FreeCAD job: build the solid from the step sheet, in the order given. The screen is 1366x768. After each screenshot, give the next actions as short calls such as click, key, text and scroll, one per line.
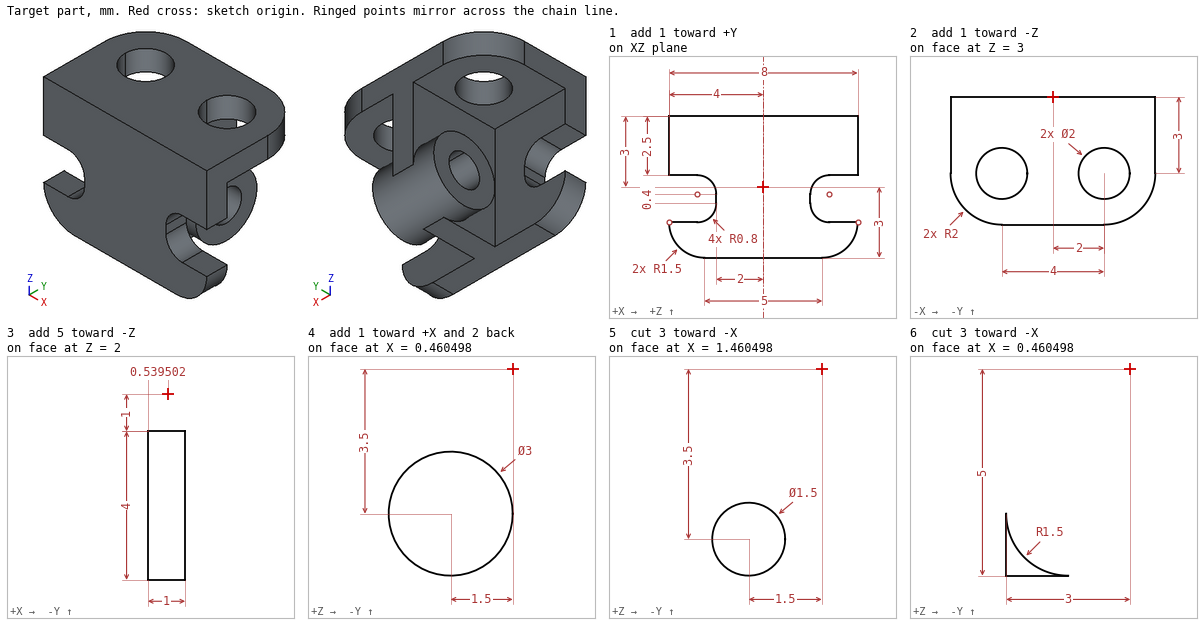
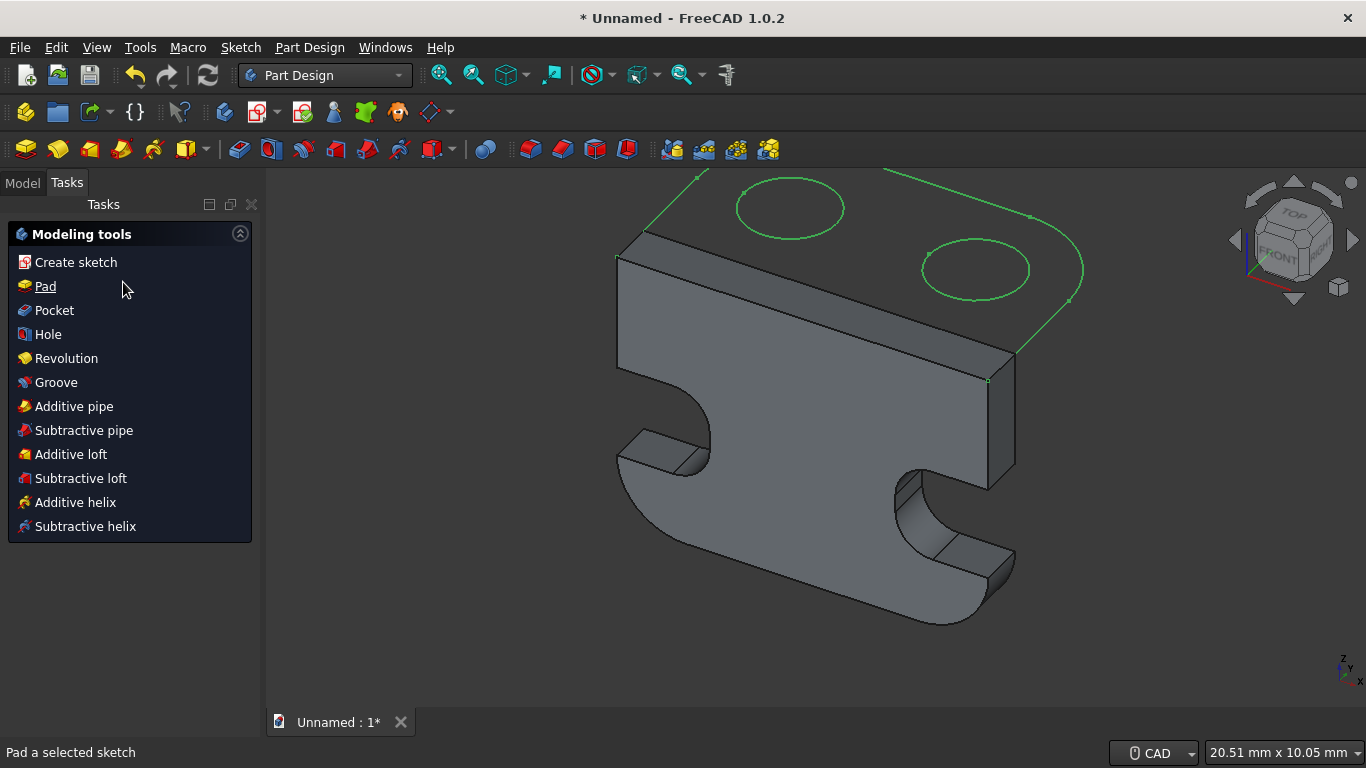
click(26, 150)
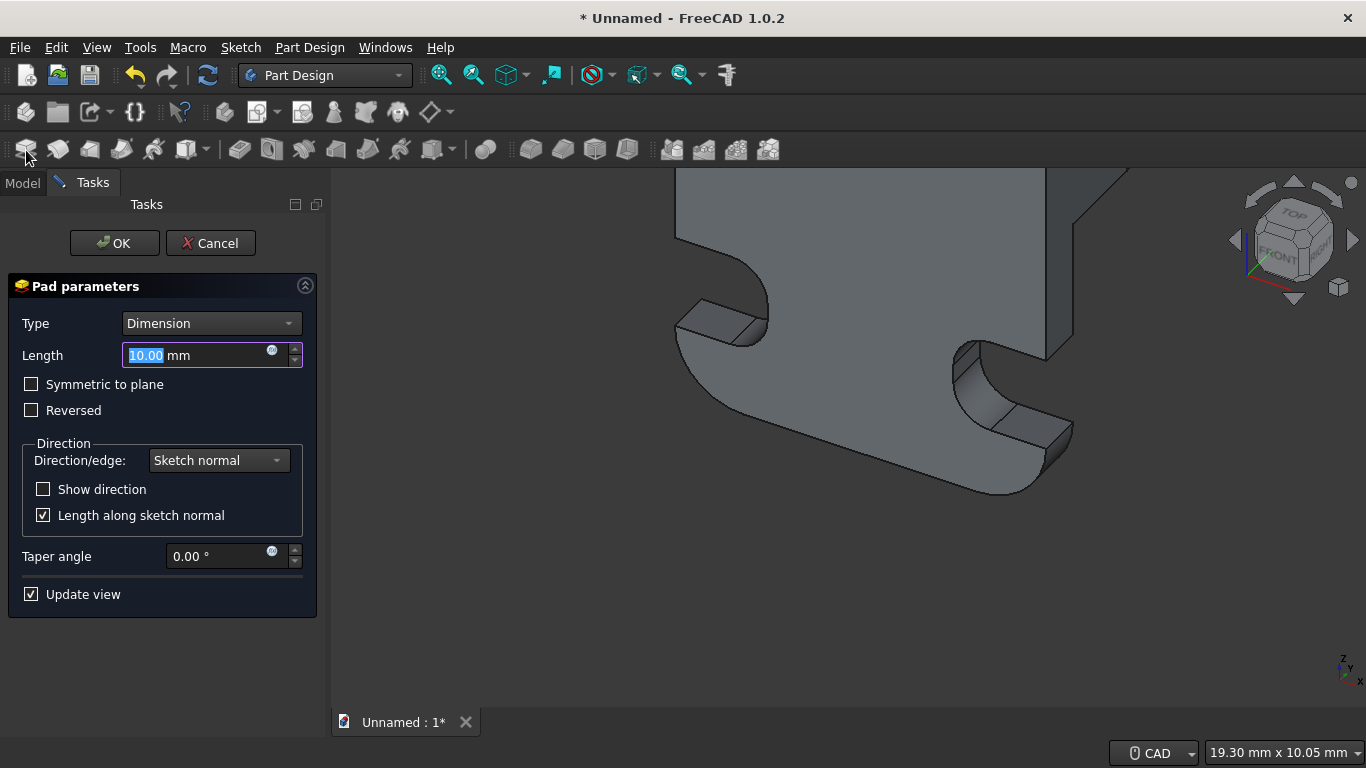
text(1)
key(Tab)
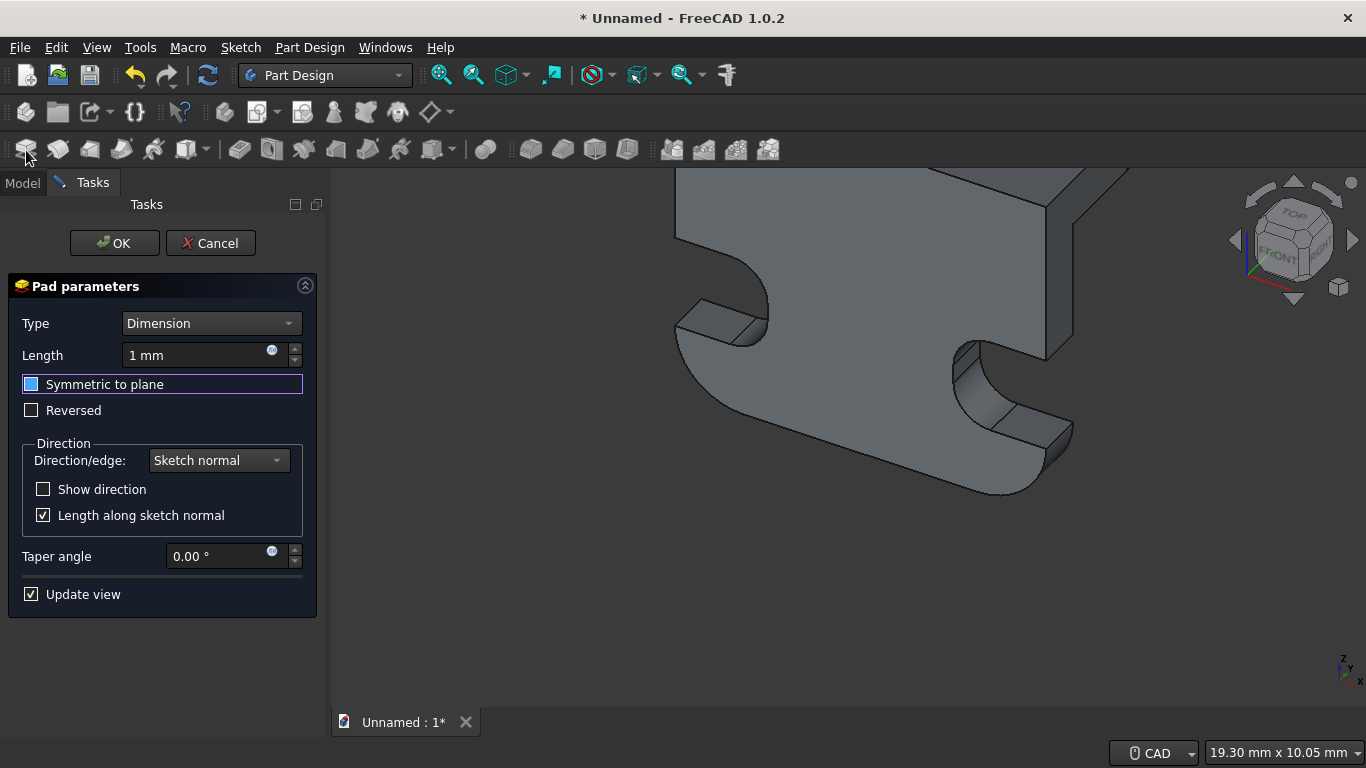
click(30, 410)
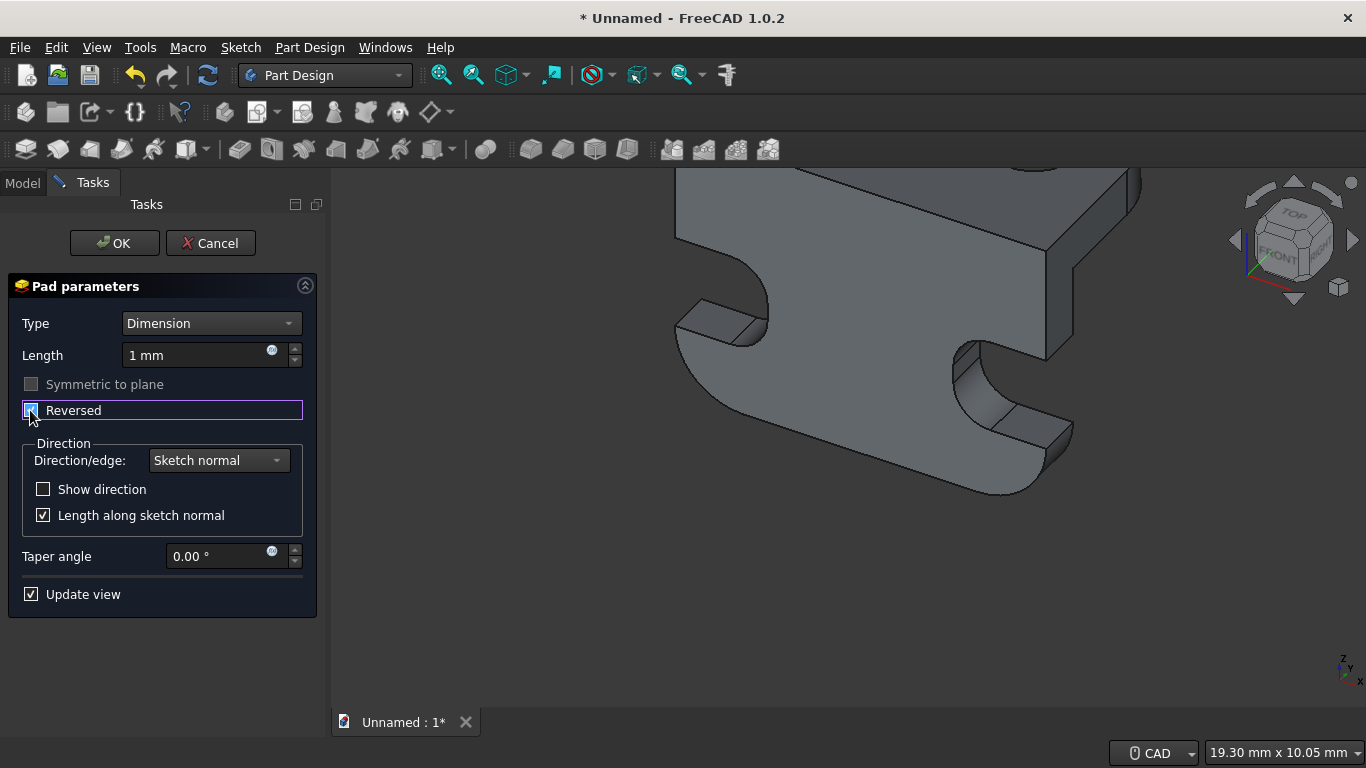
click(115, 243)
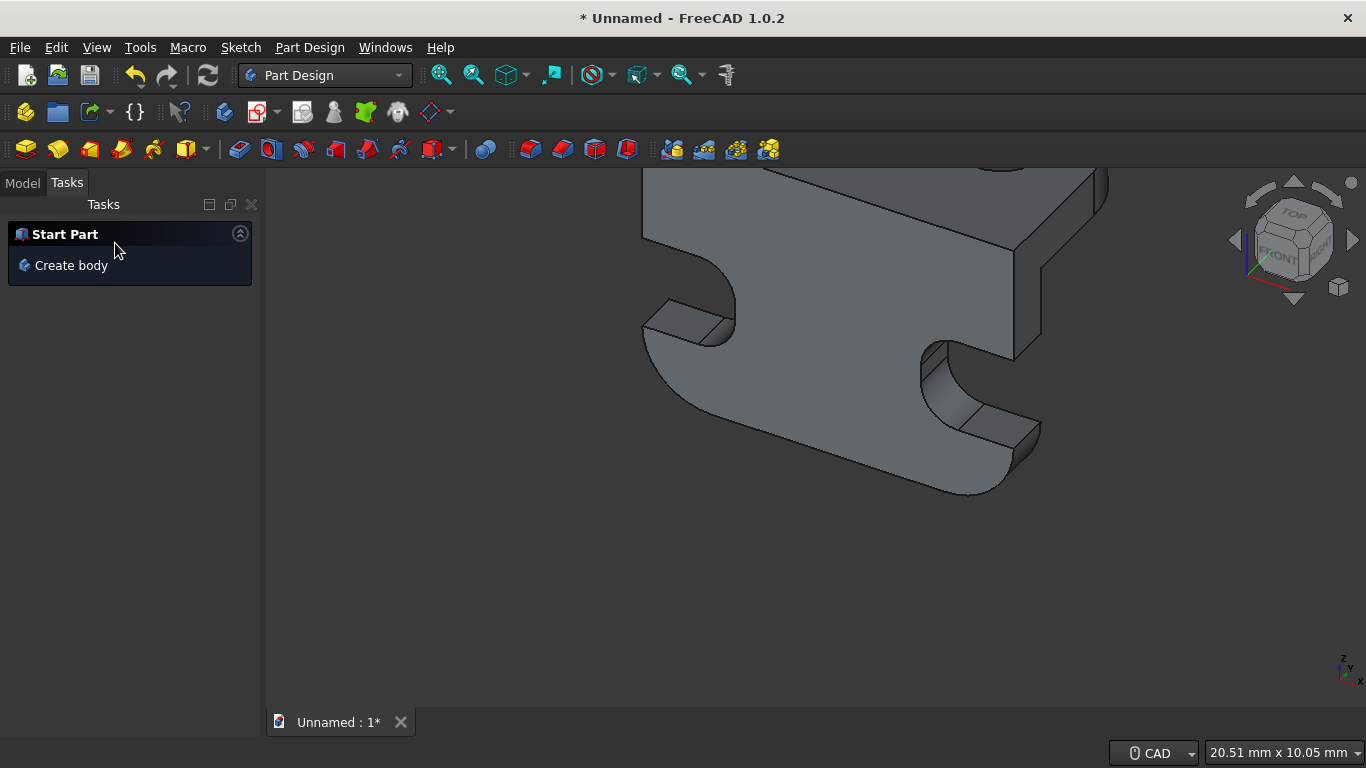
click(442, 76)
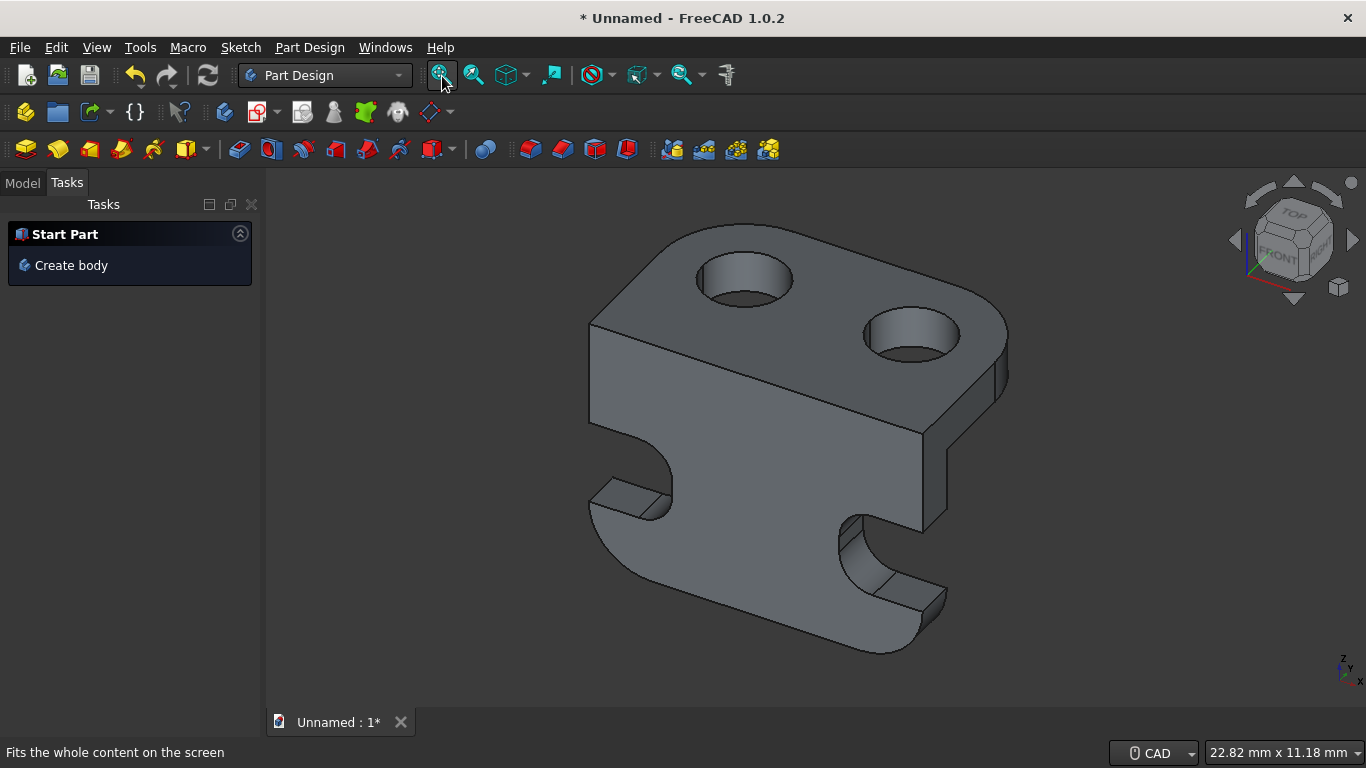
key(5)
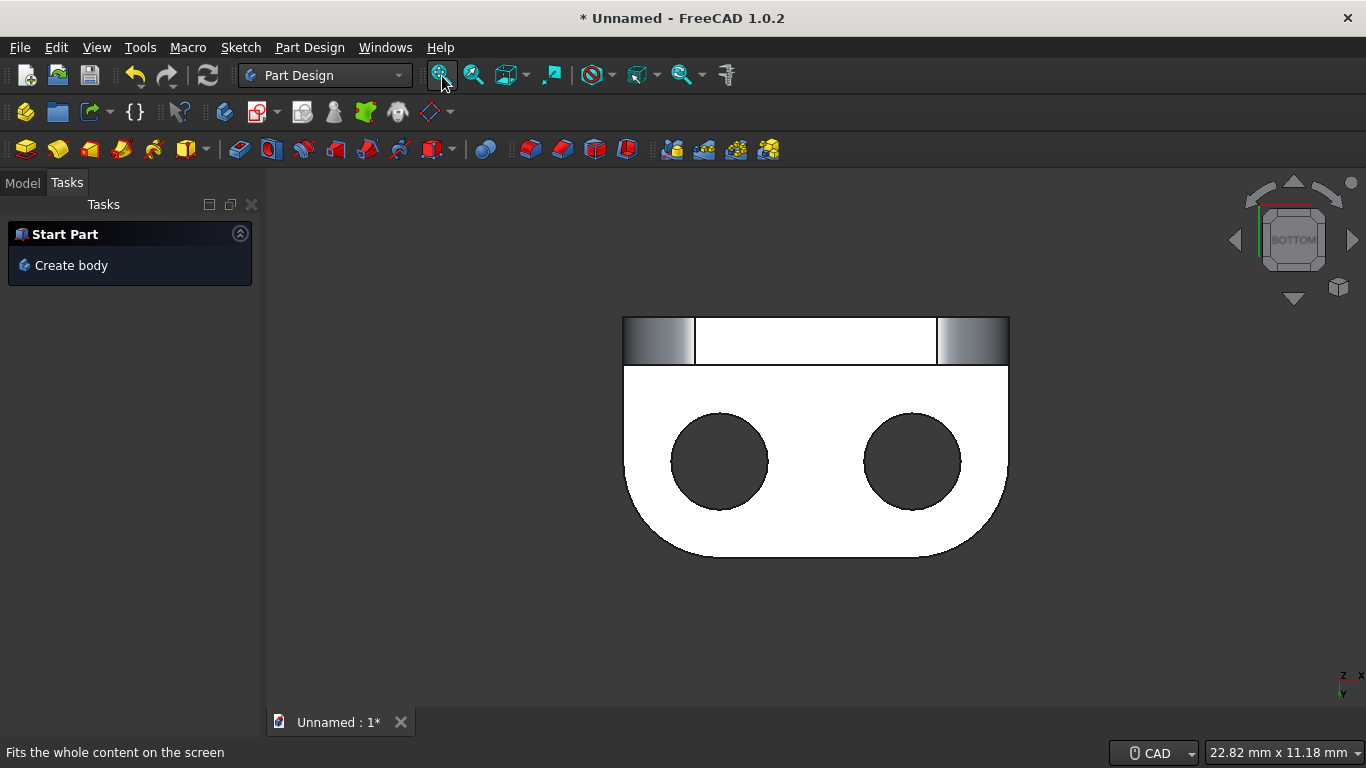
click(442, 76)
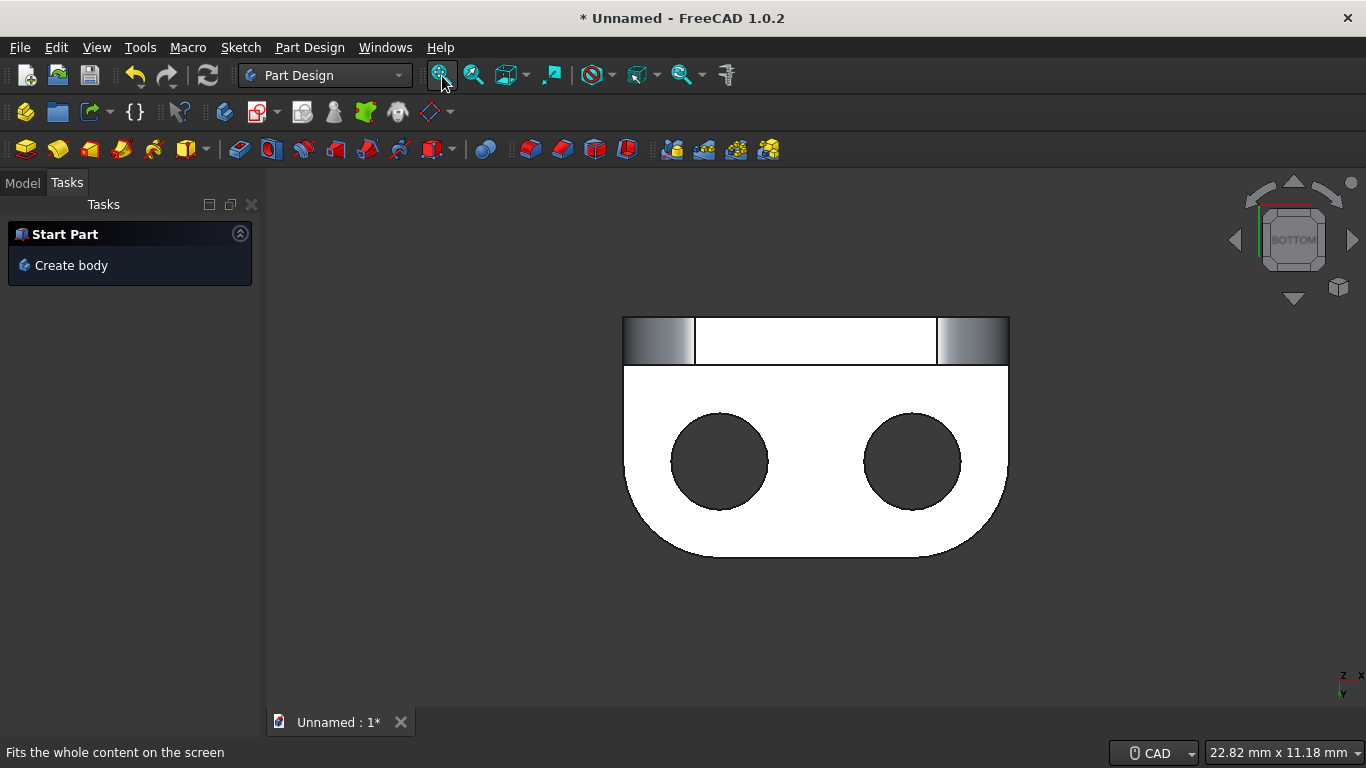
click(816, 433)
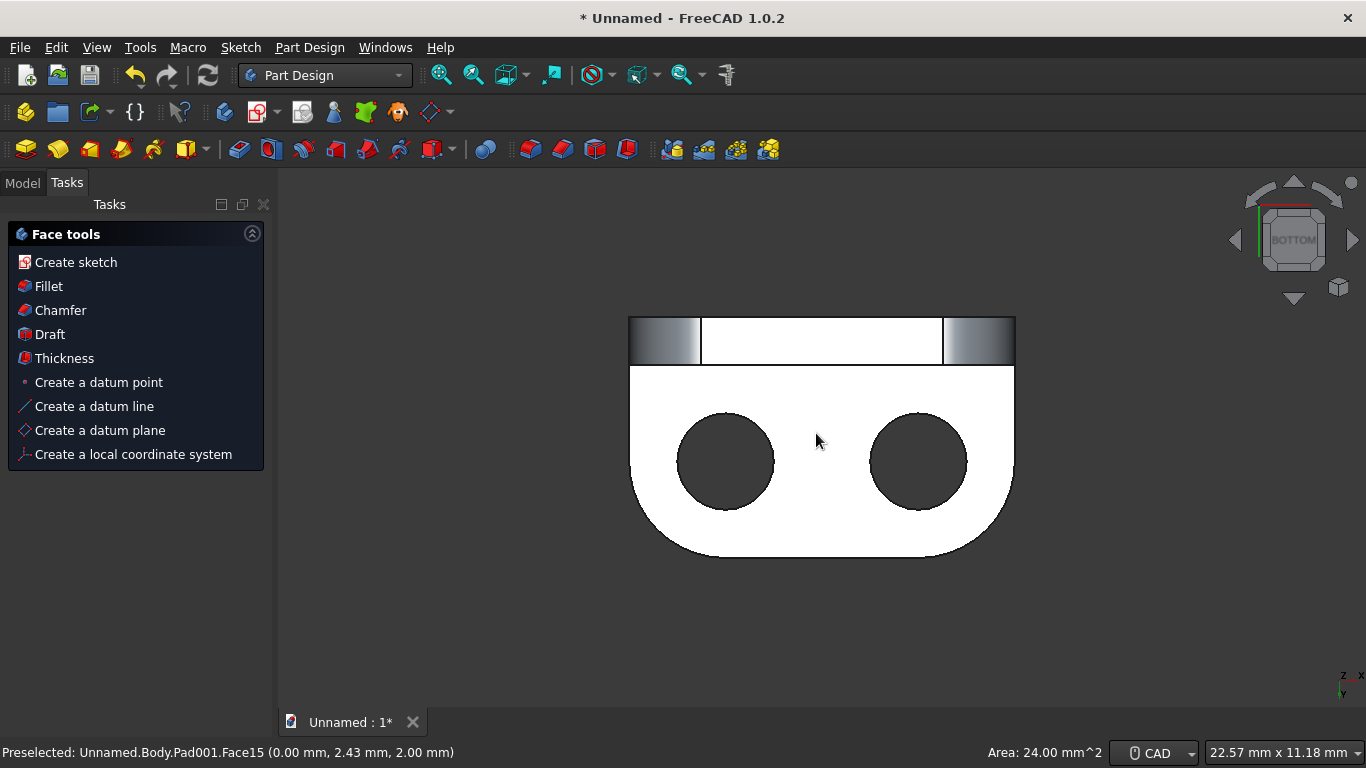
click(258, 112)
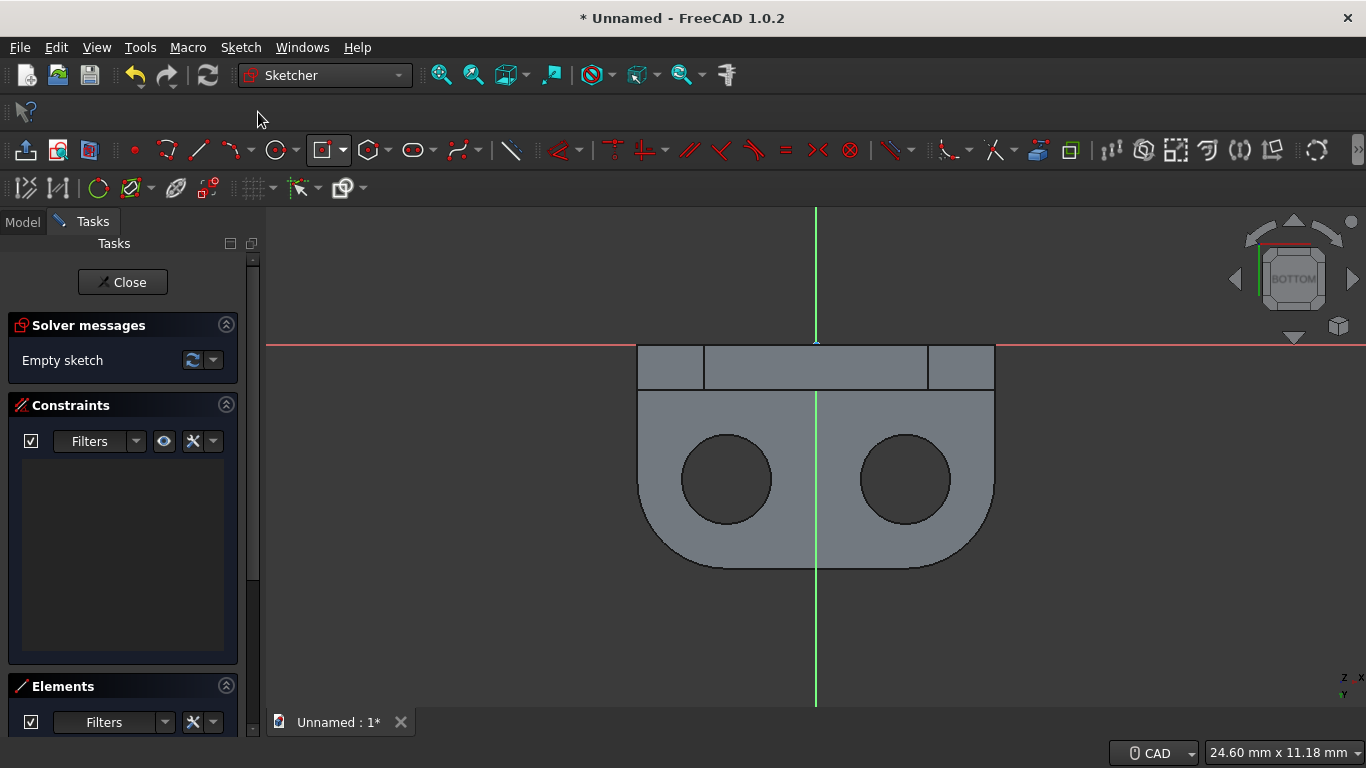
scroll(950, 457, up, 2)